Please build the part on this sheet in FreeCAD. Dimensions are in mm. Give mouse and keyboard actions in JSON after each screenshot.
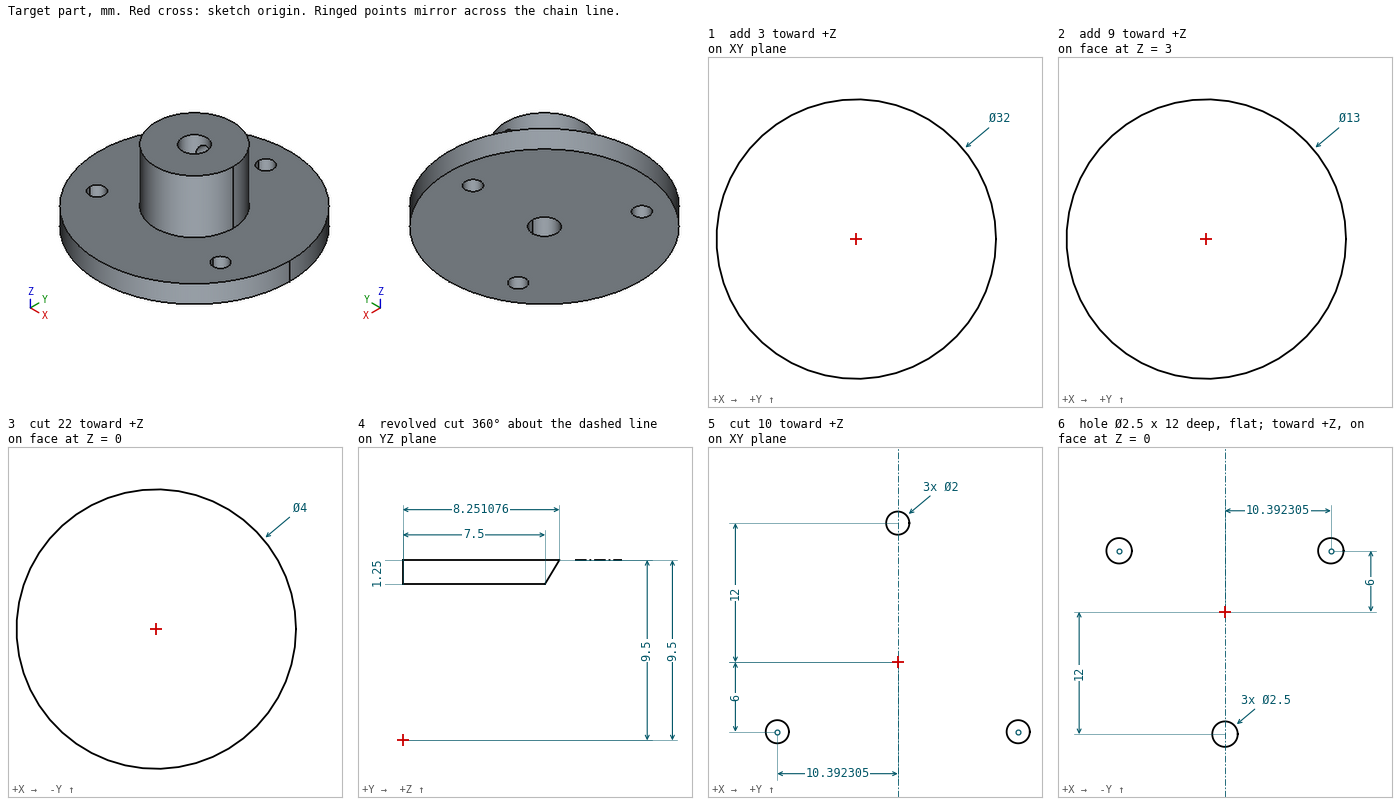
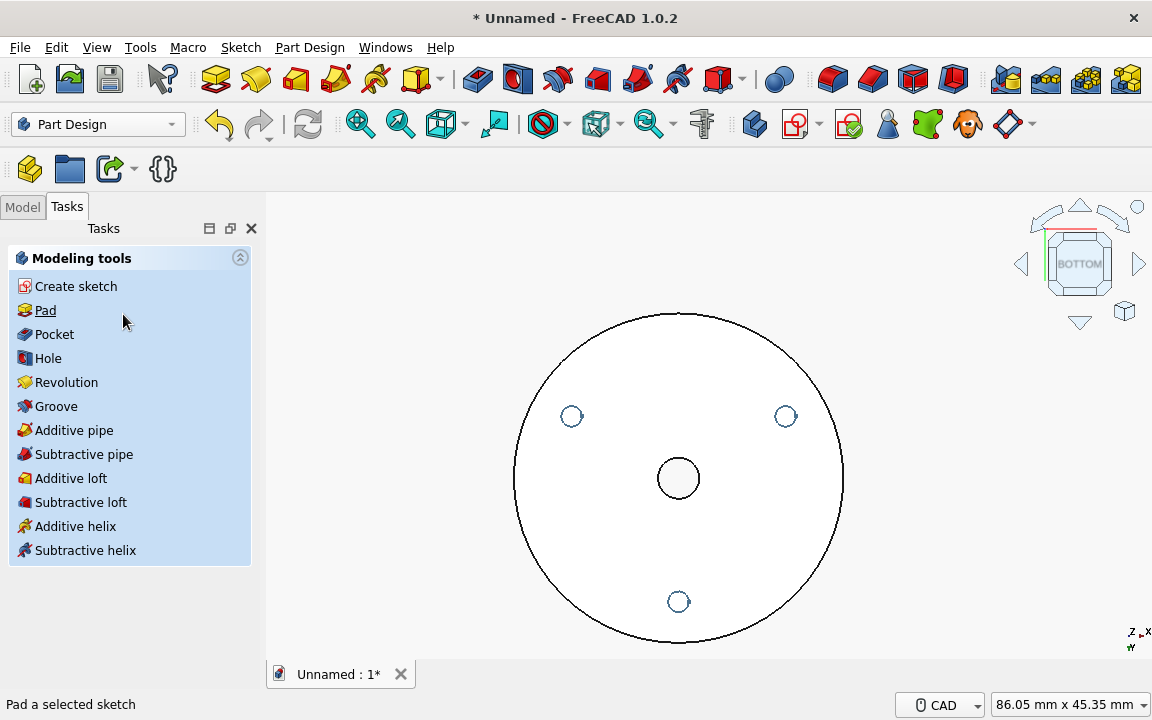
{"action": "left_click", "coordinate": [478, 80]}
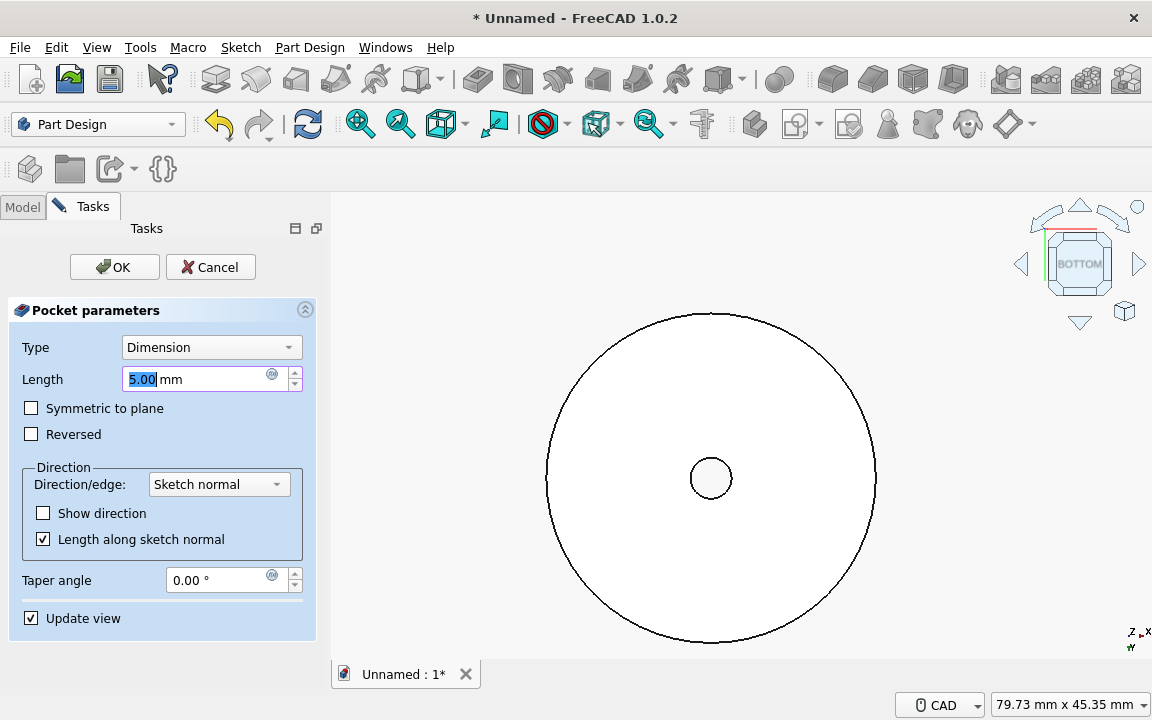
{"action": "type", "text": "10"}
{"action": "key", "text": "Tab"}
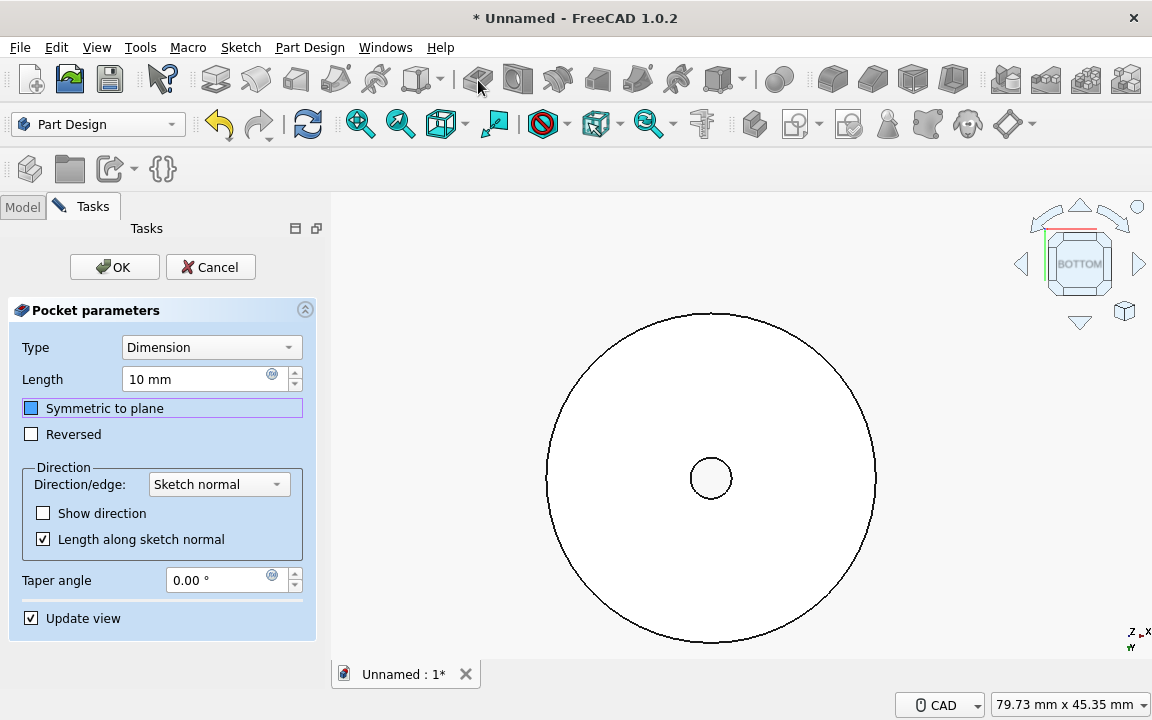
{"action": "left_click", "coordinate": [30, 434]}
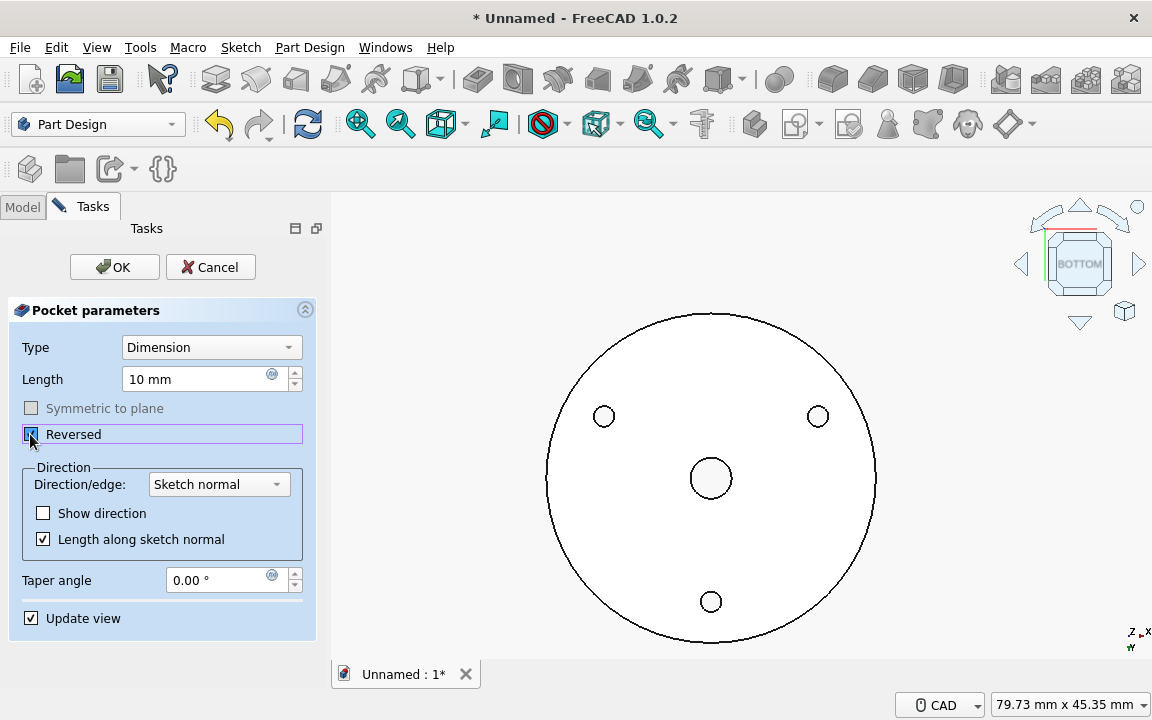
{"action": "left_click", "coordinate": [115, 267]}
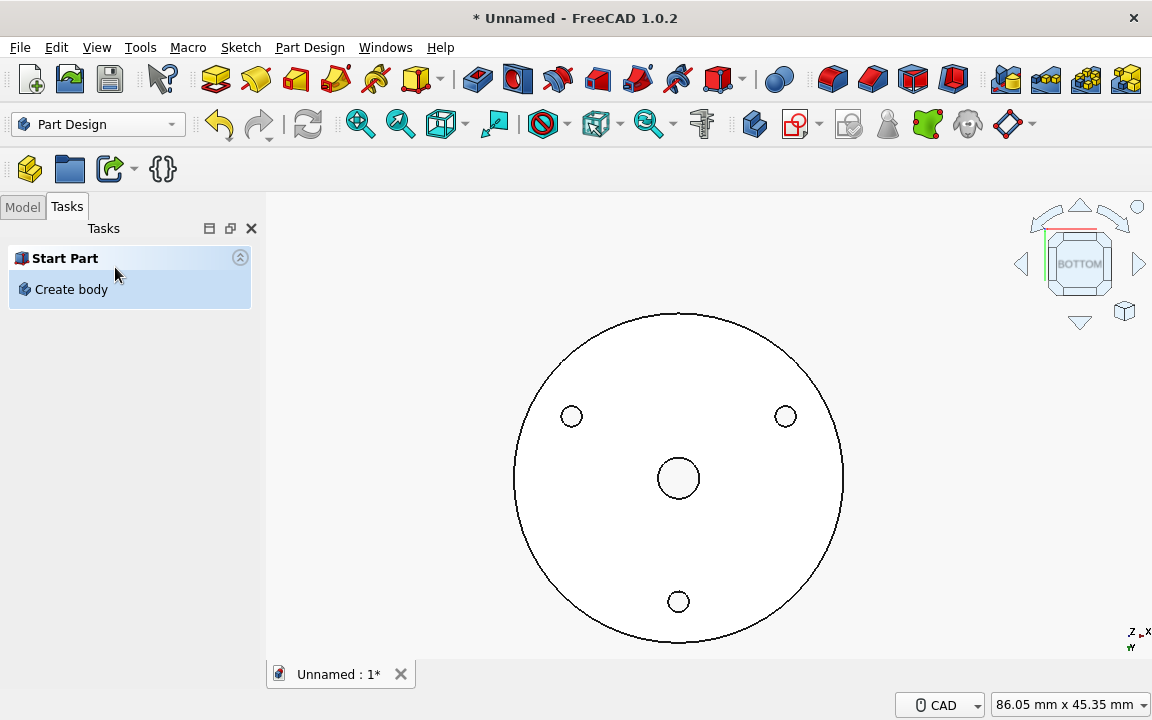
{"action": "left_click", "coordinate": [679, 383]}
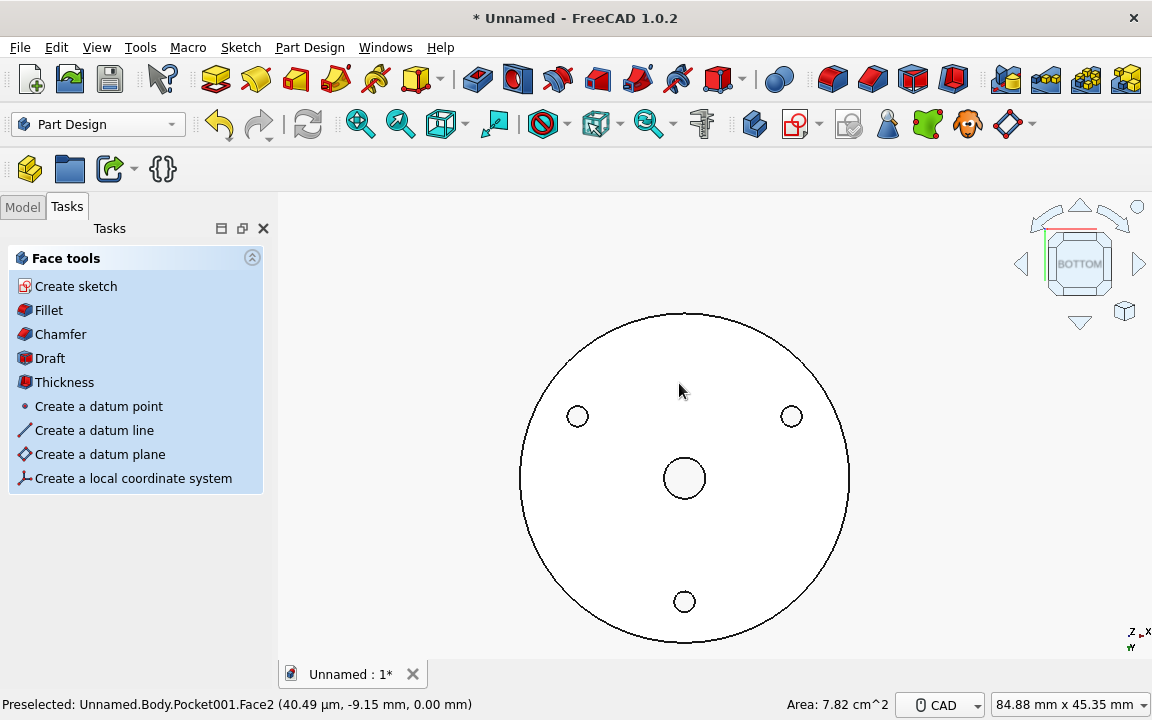
{"action": "left_click", "coordinate": [796, 124]}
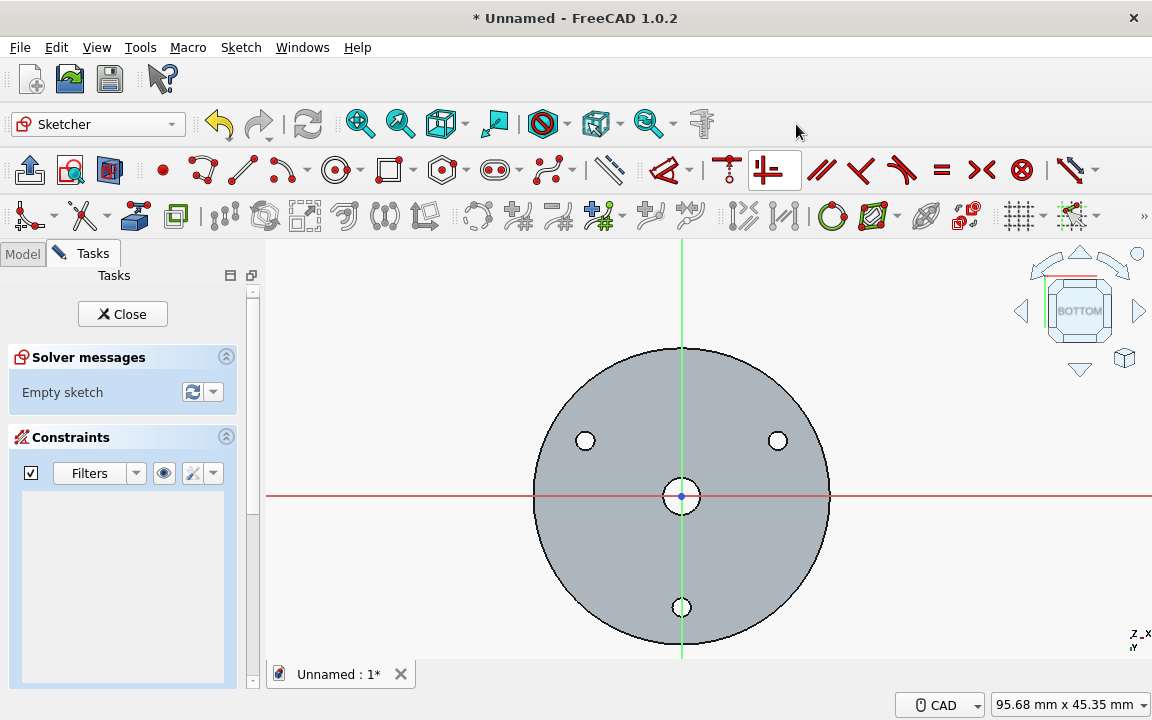
{"action": "scroll", "coordinate": [455, 267], "scroll_direction": "down", "scroll_amount": 1}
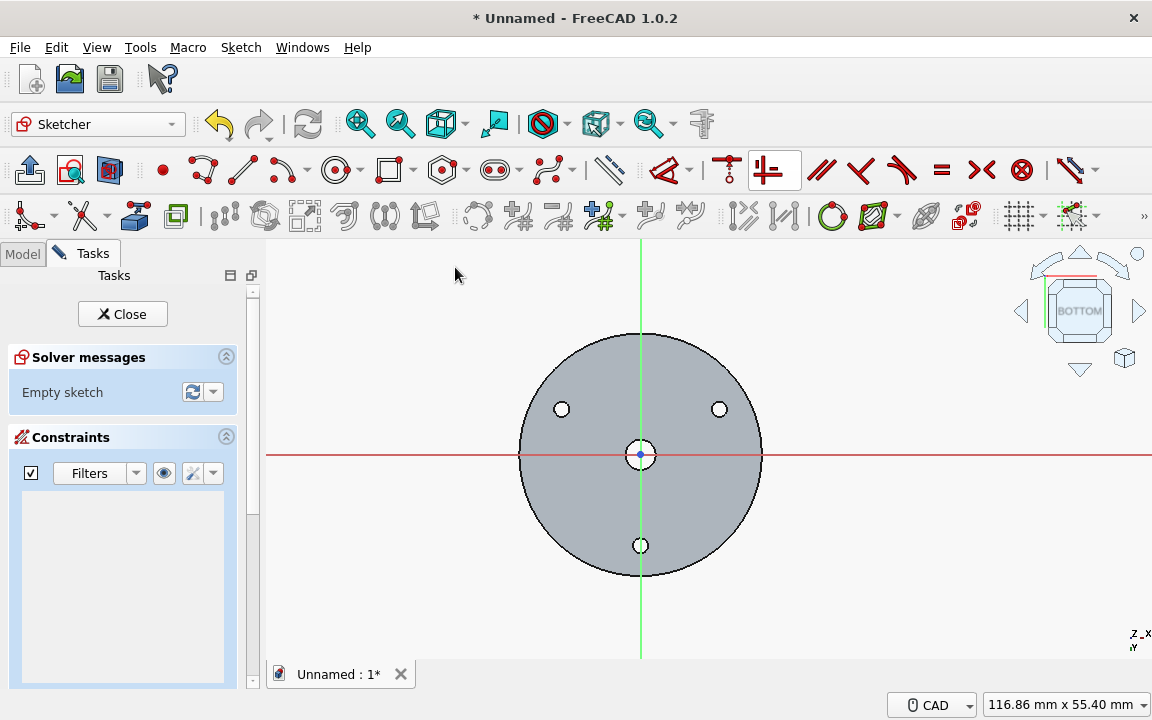
{"action": "scroll", "coordinate": [641, 512], "scroll_direction": "up", "scroll_amount": 3}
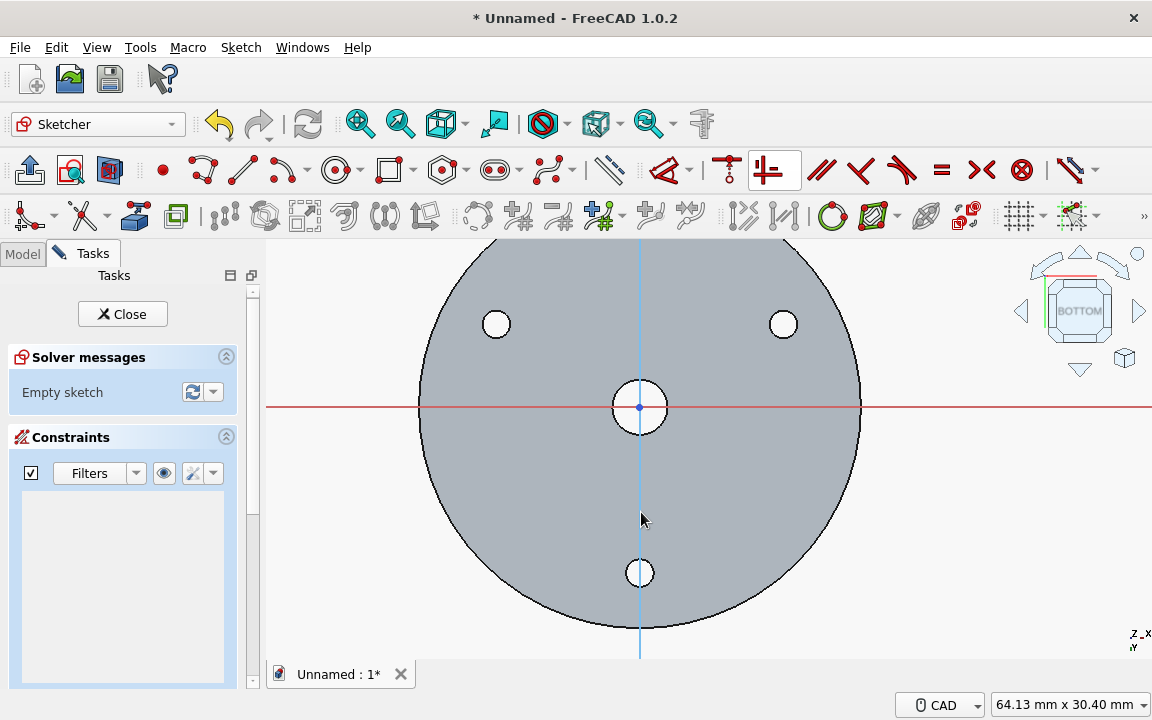
{"action": "left_click", "coordinate": [336, 170]}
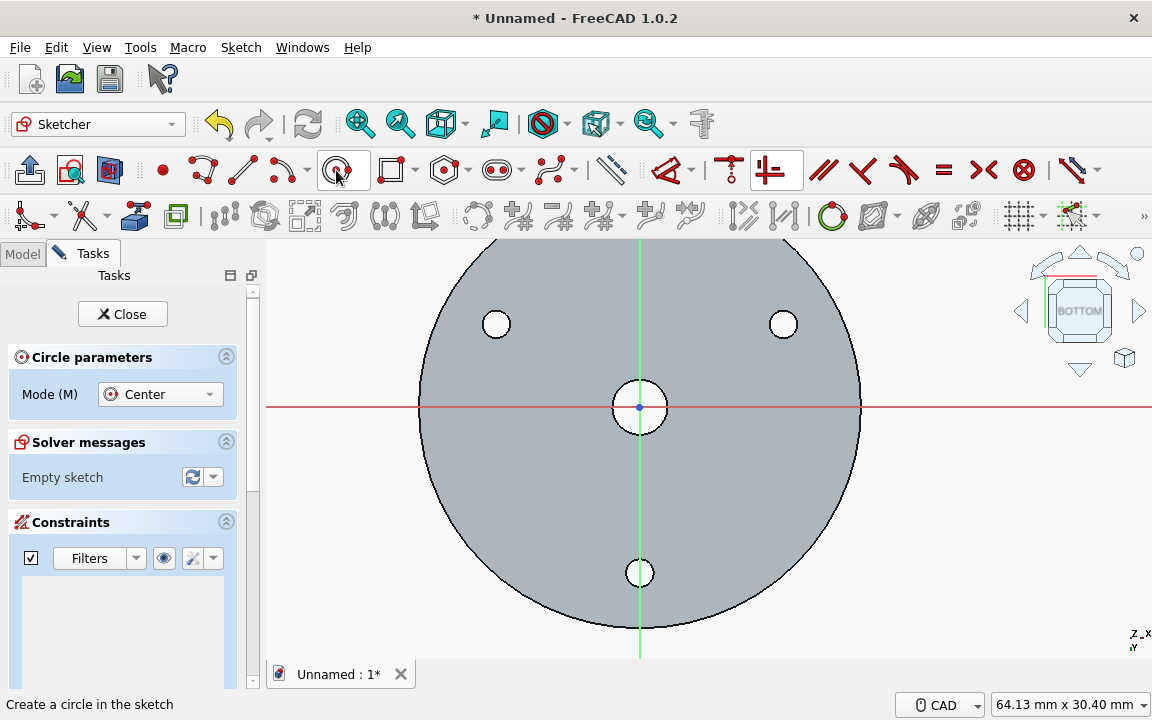
{"action": "scroll", "coordinate": [640, 573], "scroll_direction": "up", "scroll_amount": 2}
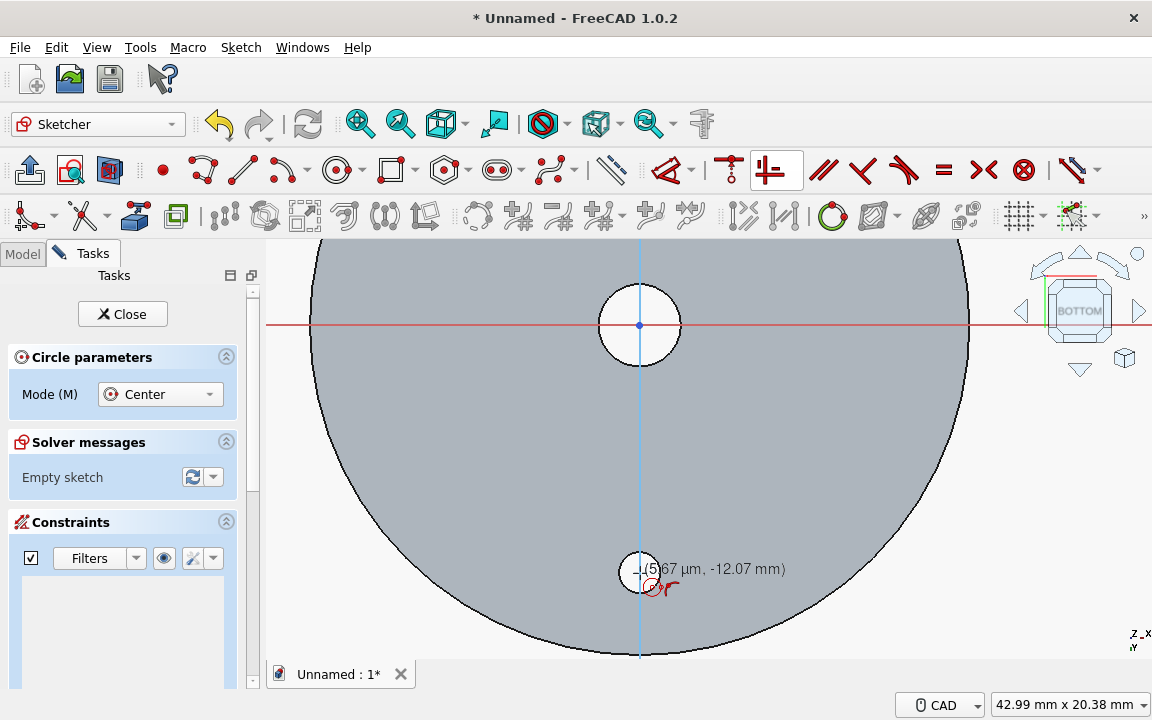
{"action": "left_click", "coordinate": [640, 573]}
{"action": "mouse_move", "coordinate": [658, 554]}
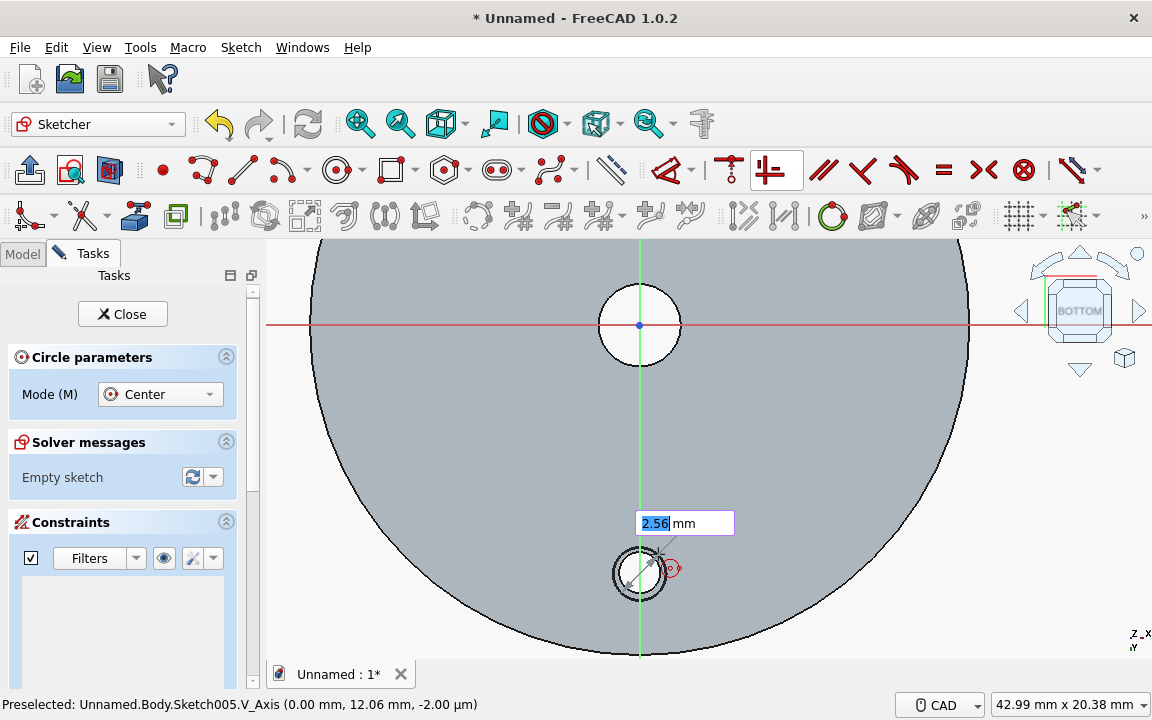
{"action": "type", "text": "2.5"}
{"action": "key", "text": "Return"}